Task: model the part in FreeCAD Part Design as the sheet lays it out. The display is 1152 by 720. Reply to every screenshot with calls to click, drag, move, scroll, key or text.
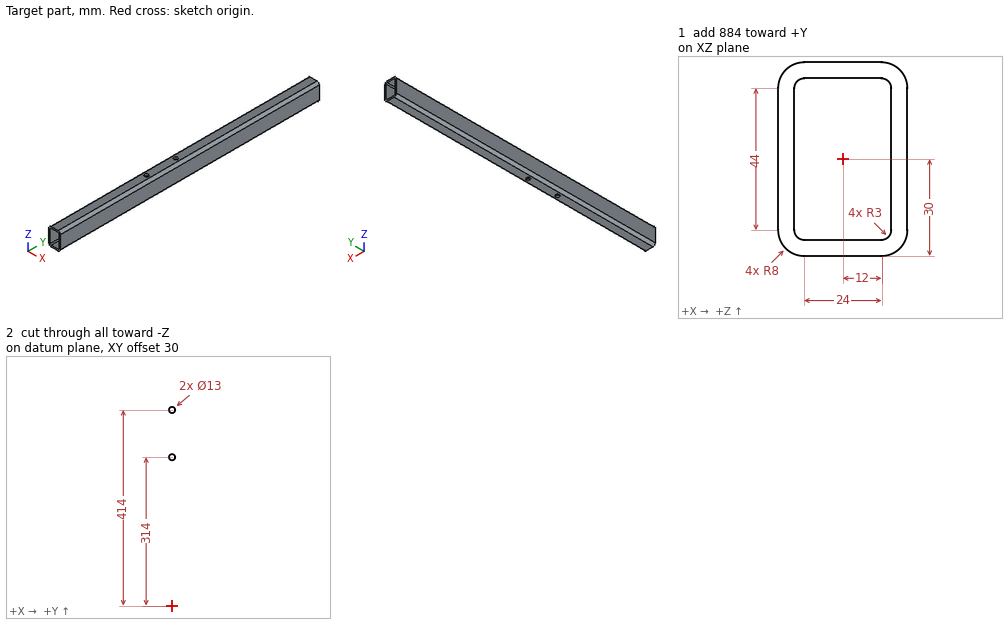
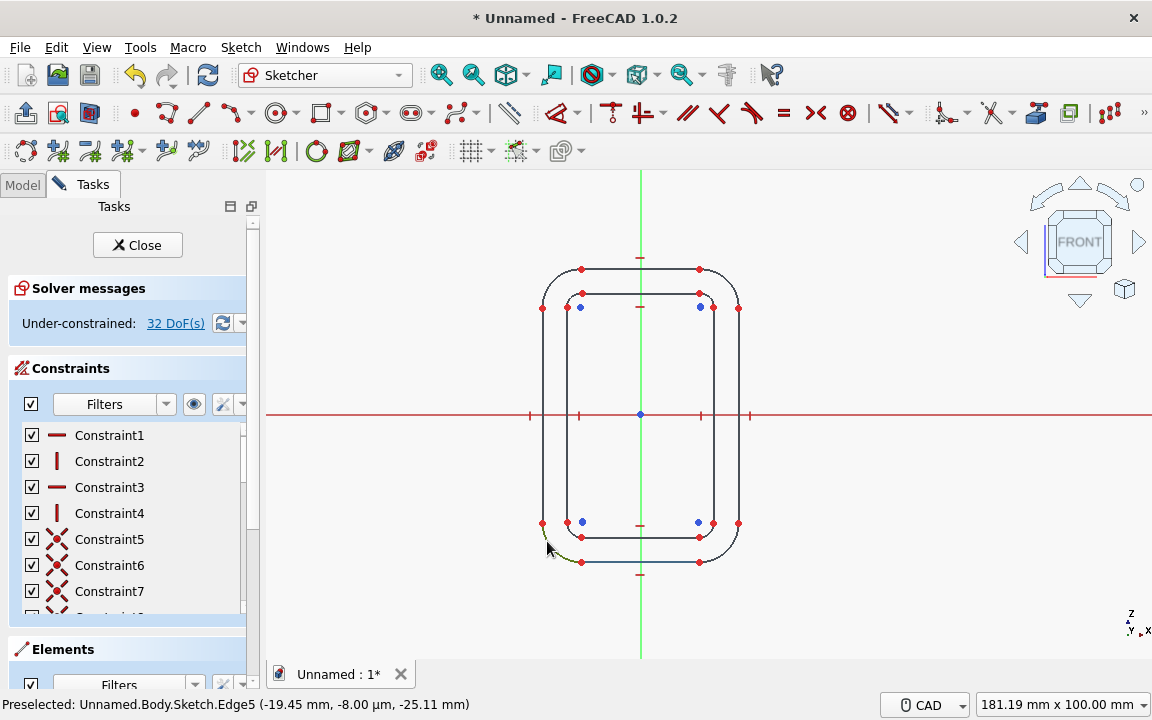
key(t)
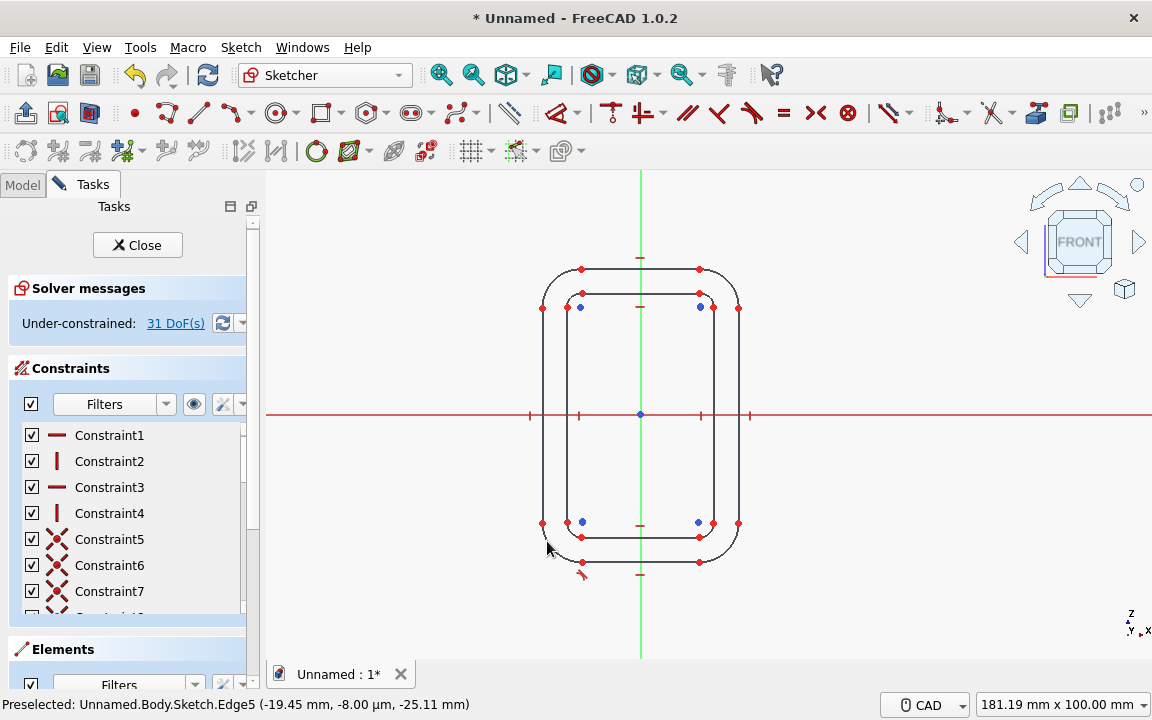
click(664, 562)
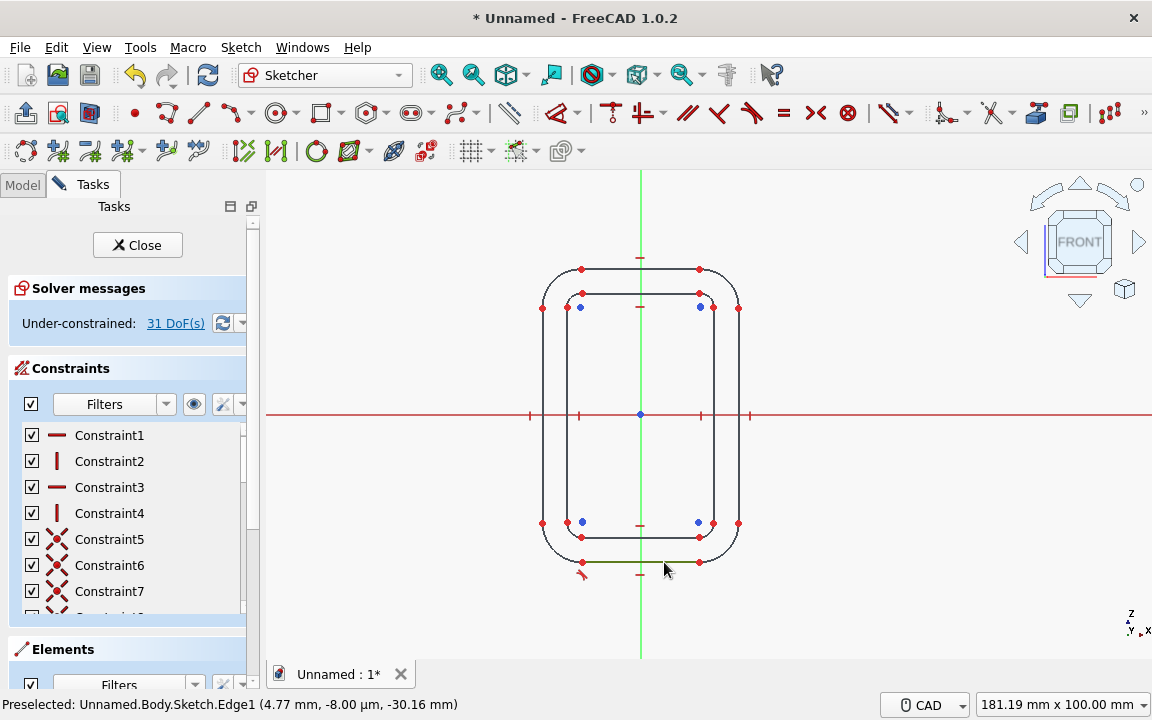
click(717, 558)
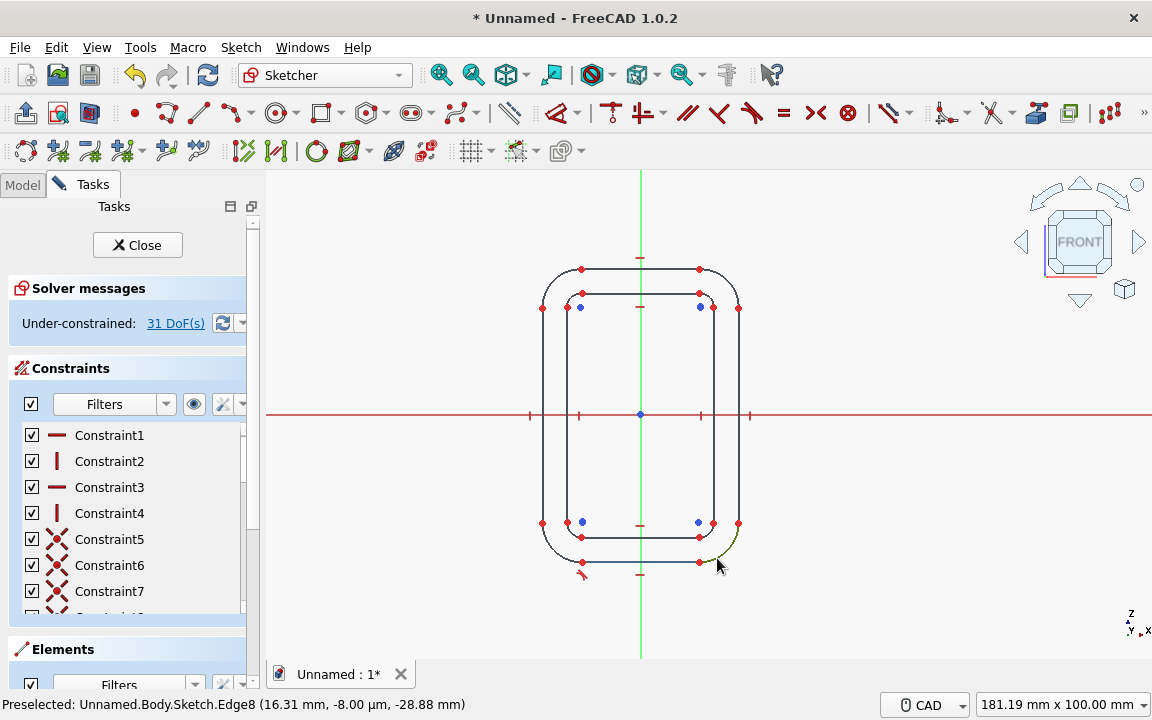
click(752, 114)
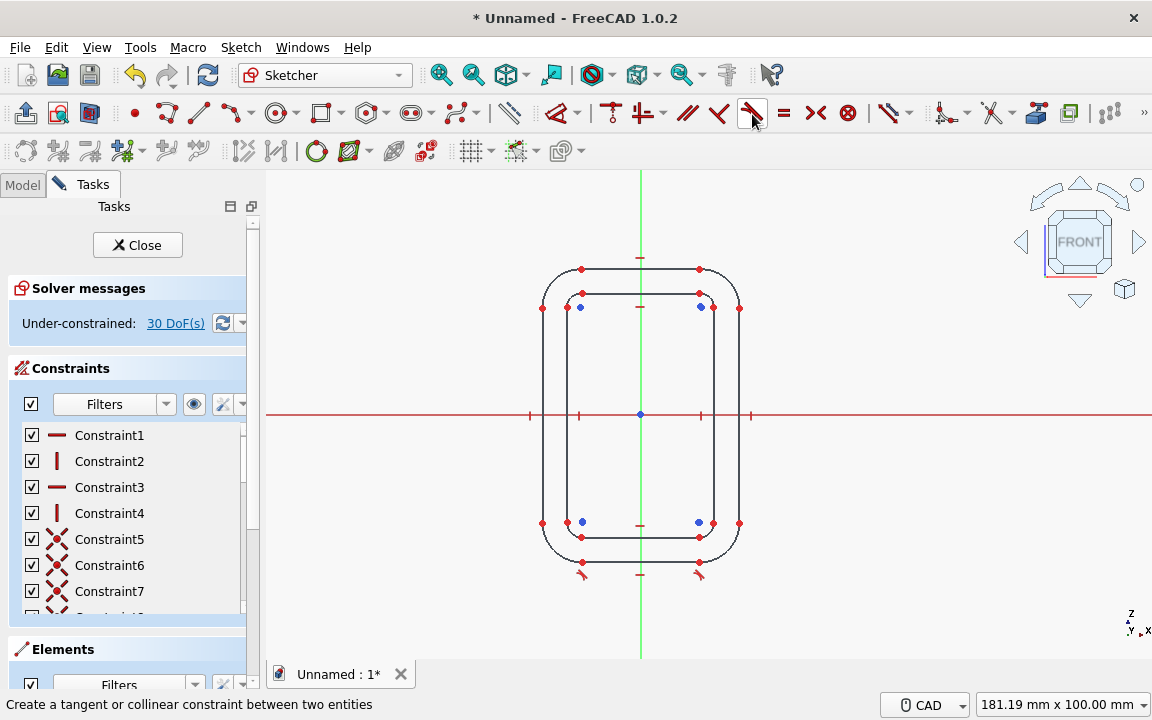
click(543, 459)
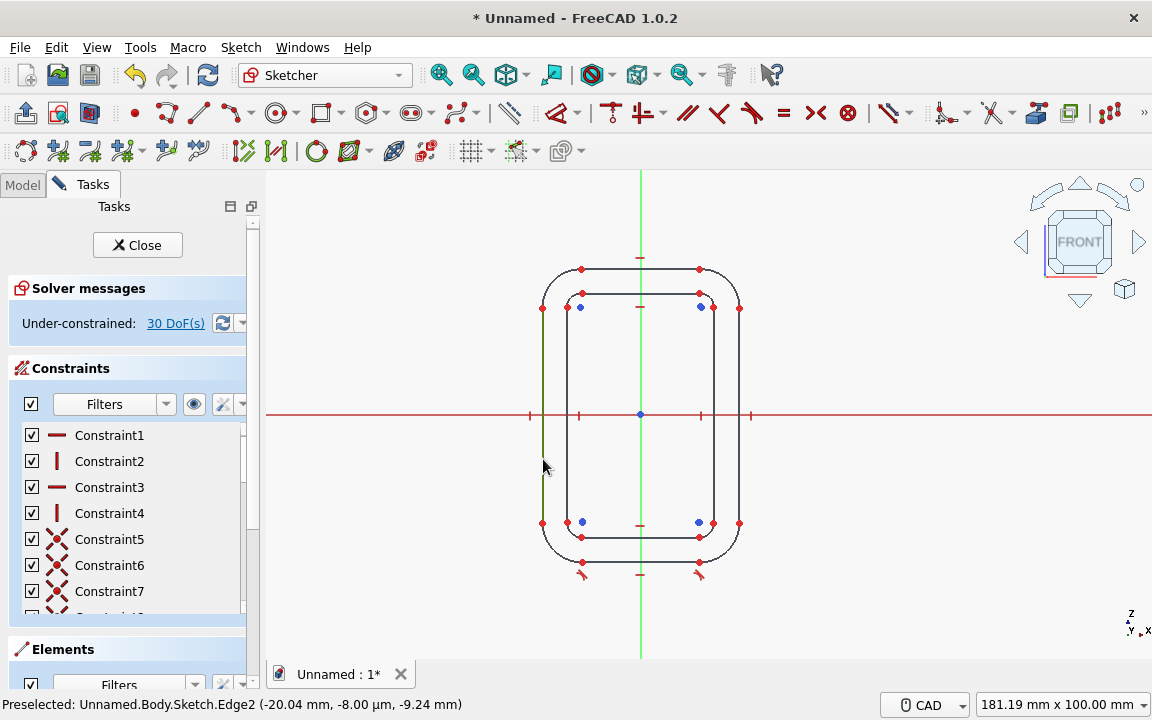
click(547, 541)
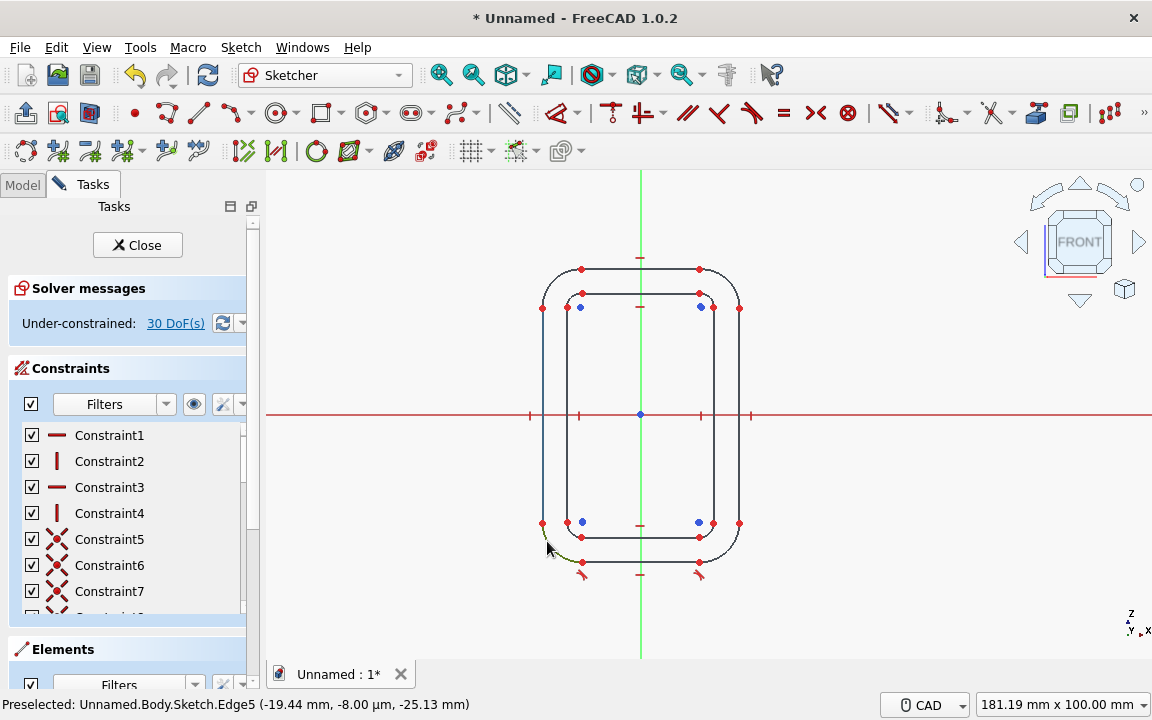
key(t)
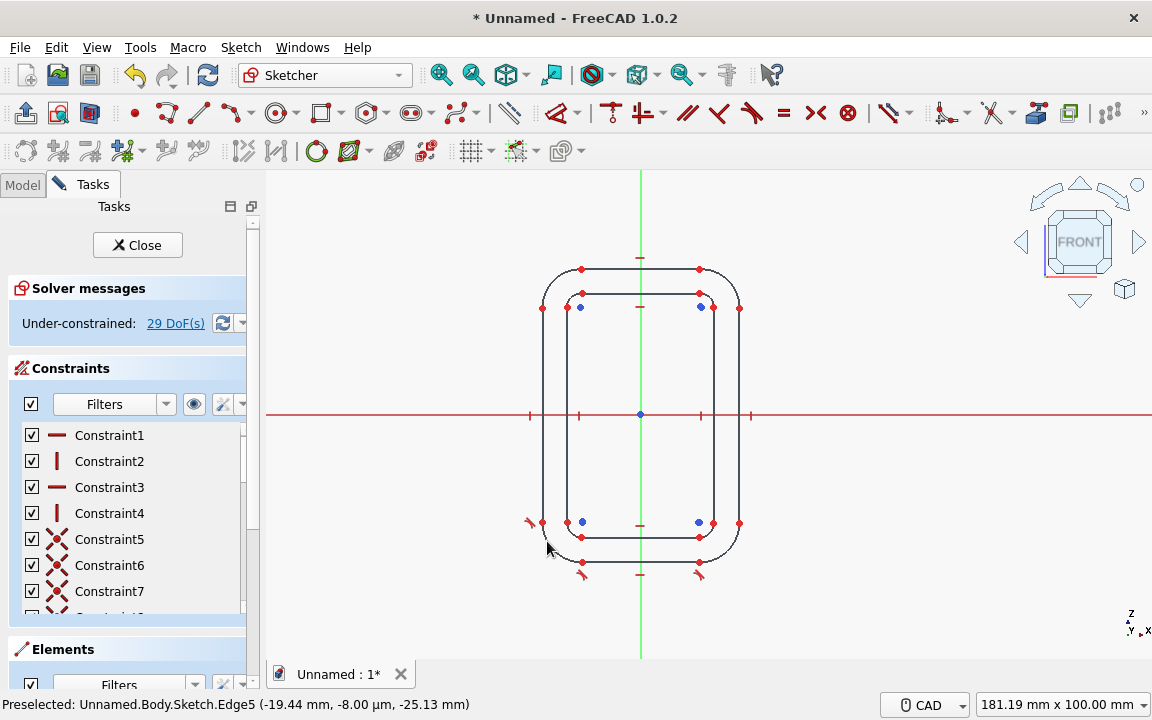
click(543, 458)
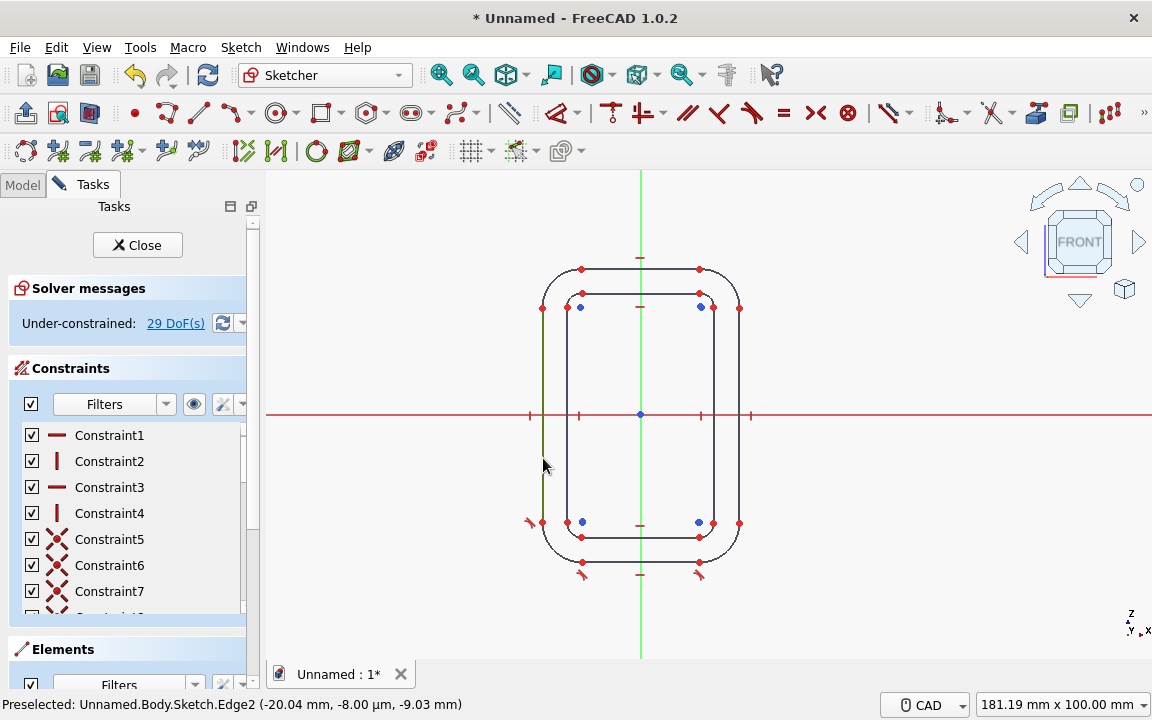
click(564, 273)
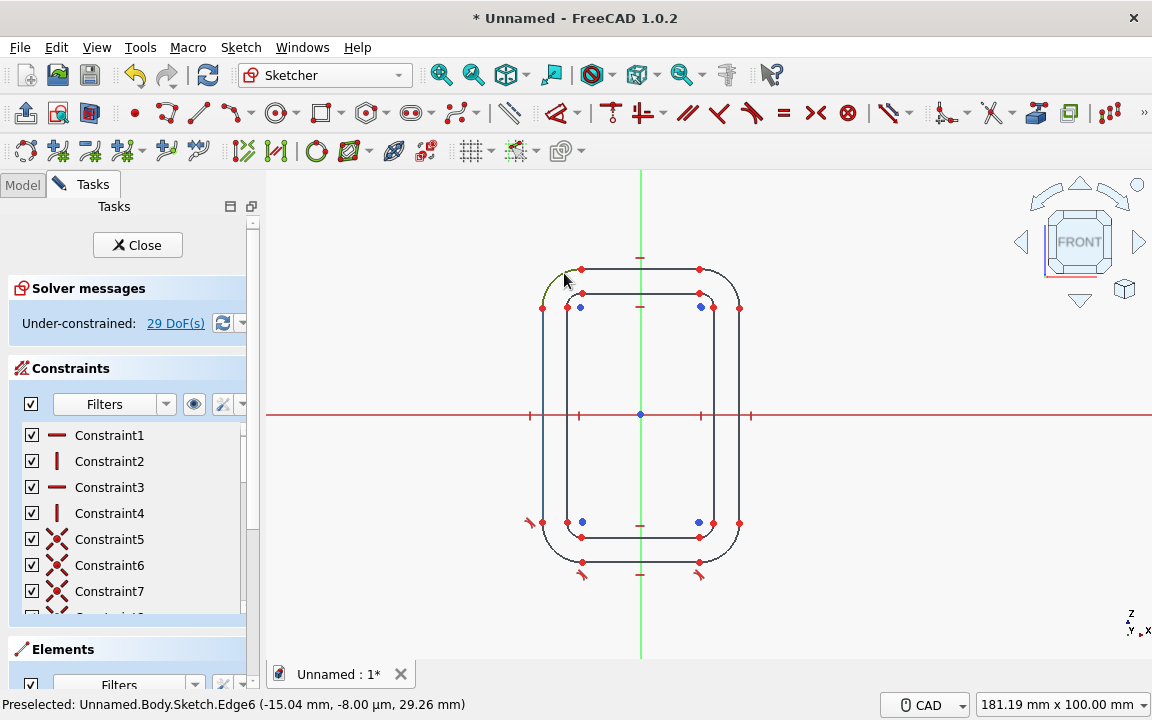
click(752, 114)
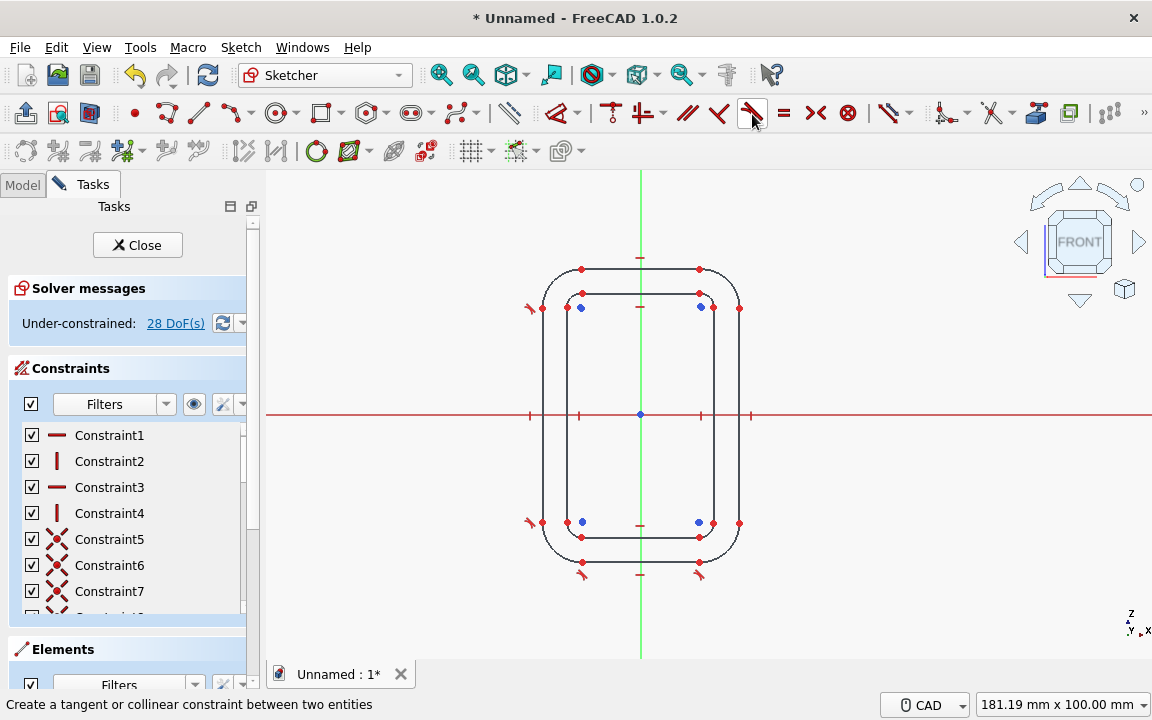
click(617, 269)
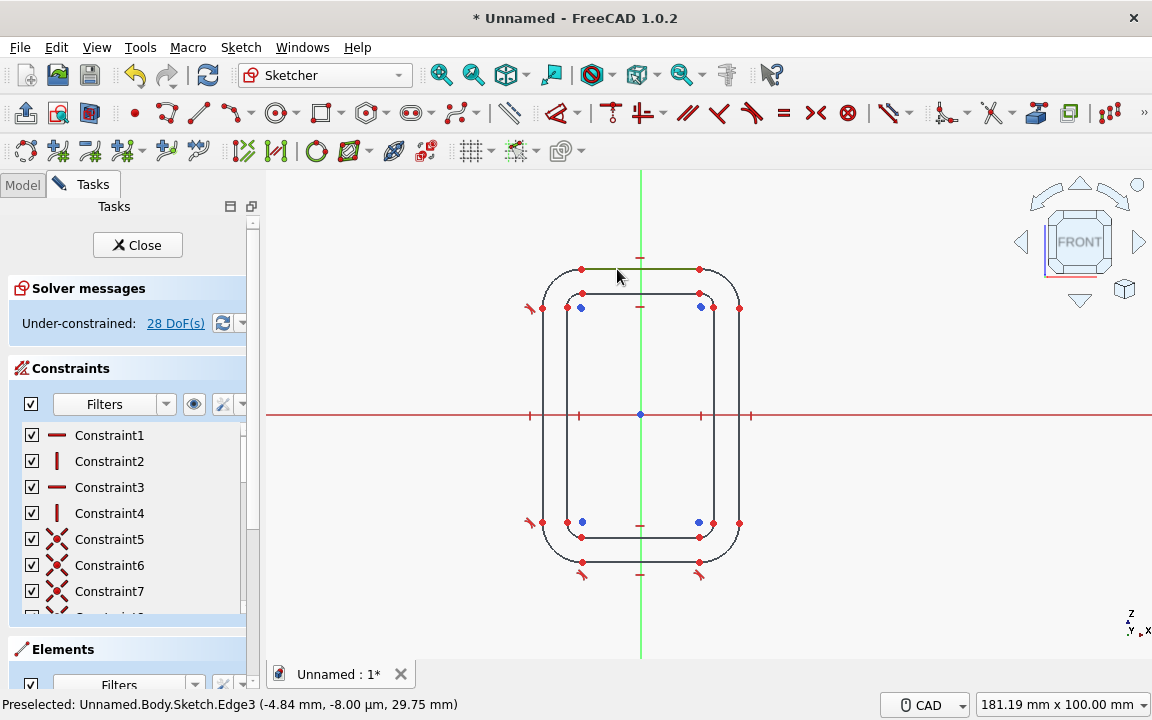
click(564, 274)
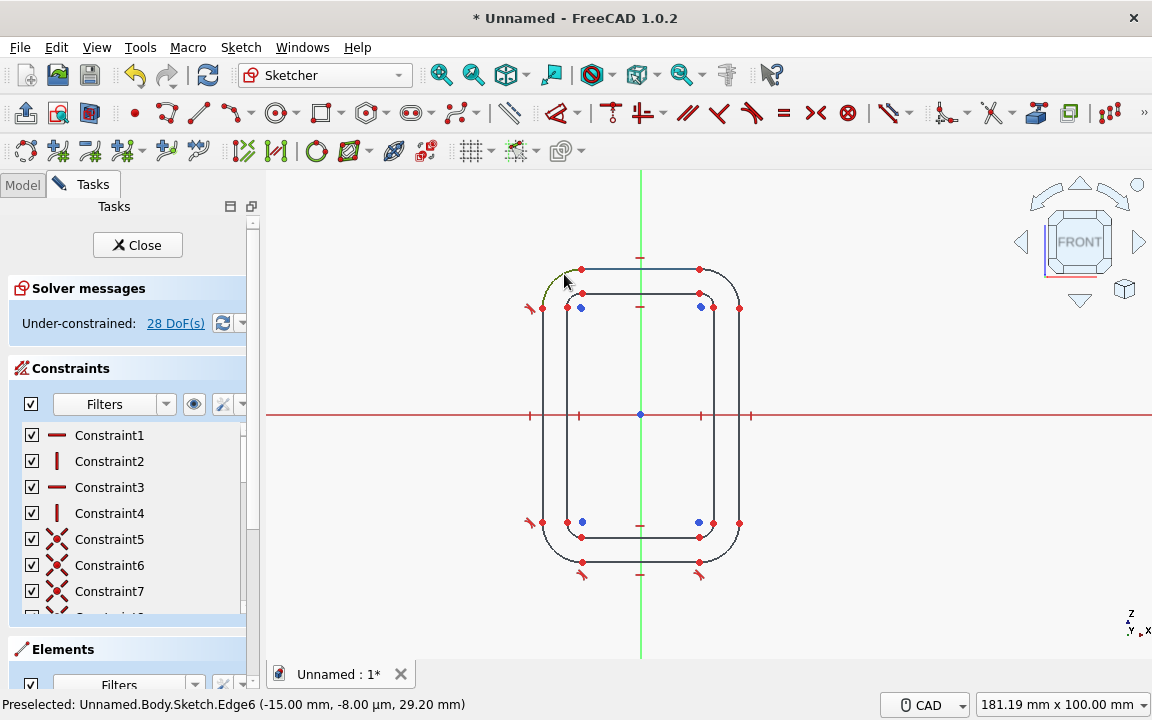
click(752, 114)